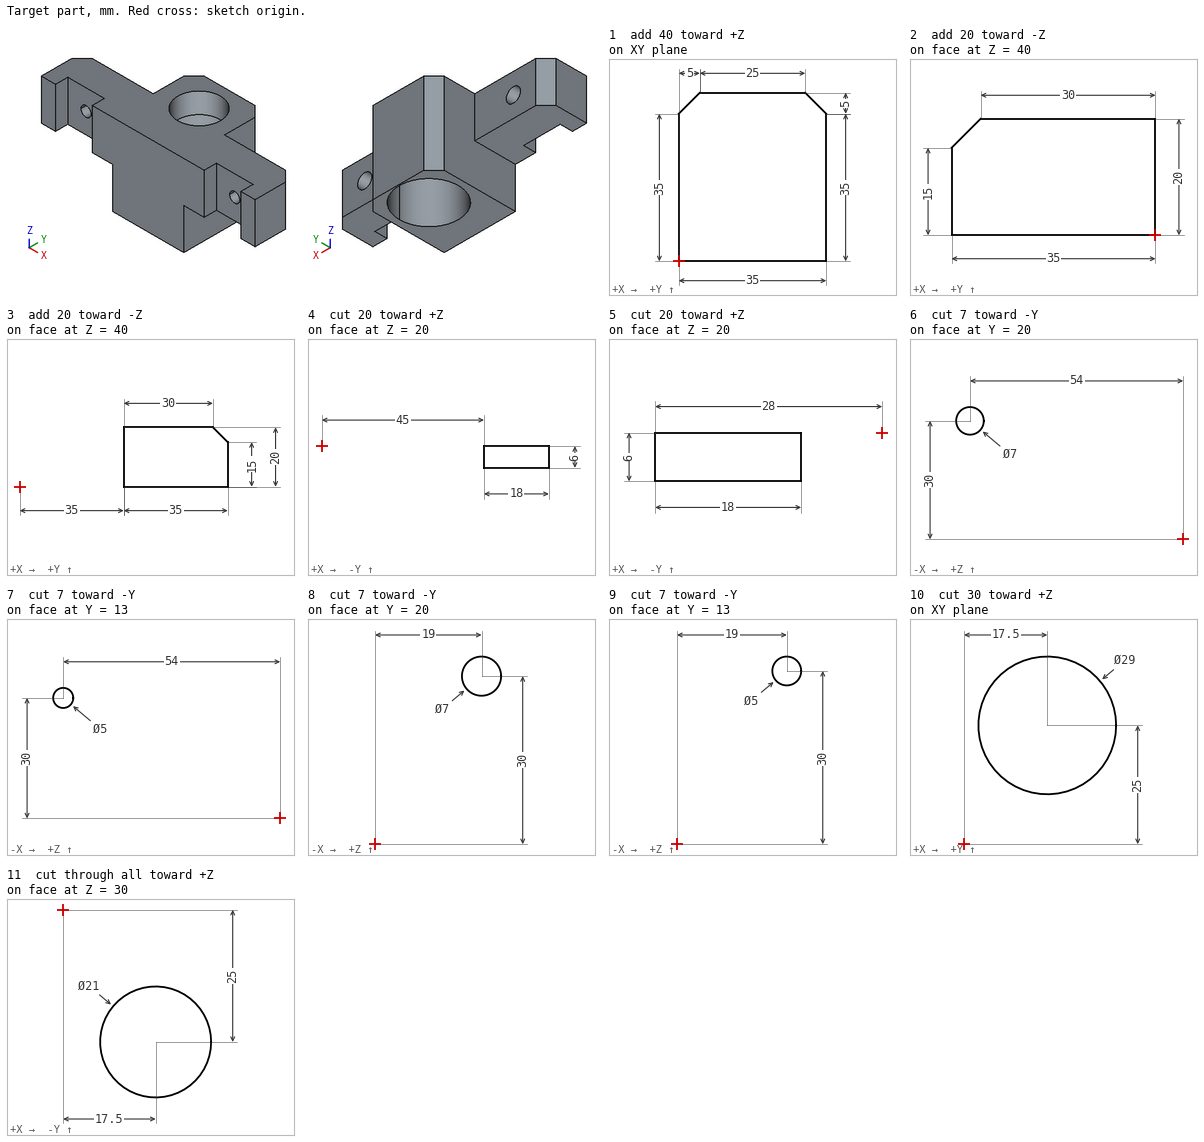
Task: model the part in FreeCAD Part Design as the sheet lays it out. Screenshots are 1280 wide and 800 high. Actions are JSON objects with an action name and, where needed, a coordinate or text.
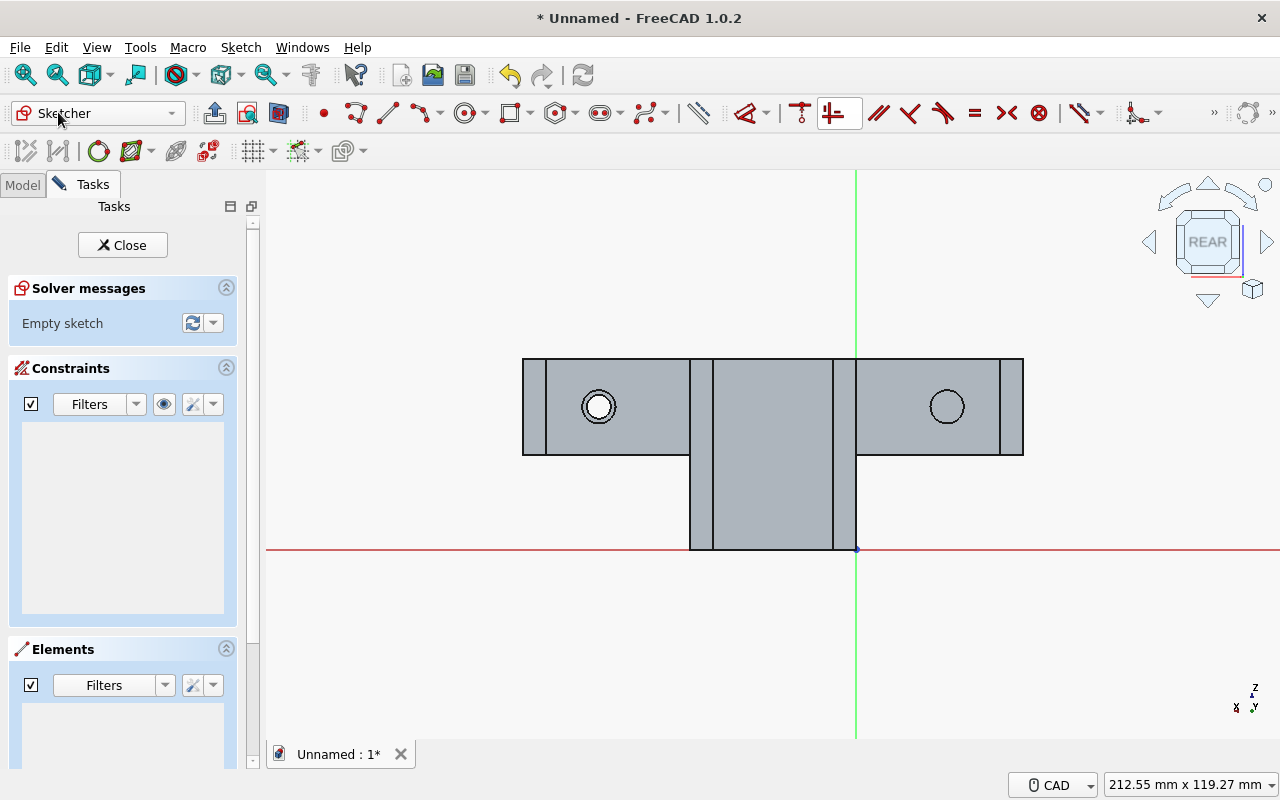
{"action": "left_click", "coordinate": [280, 114]}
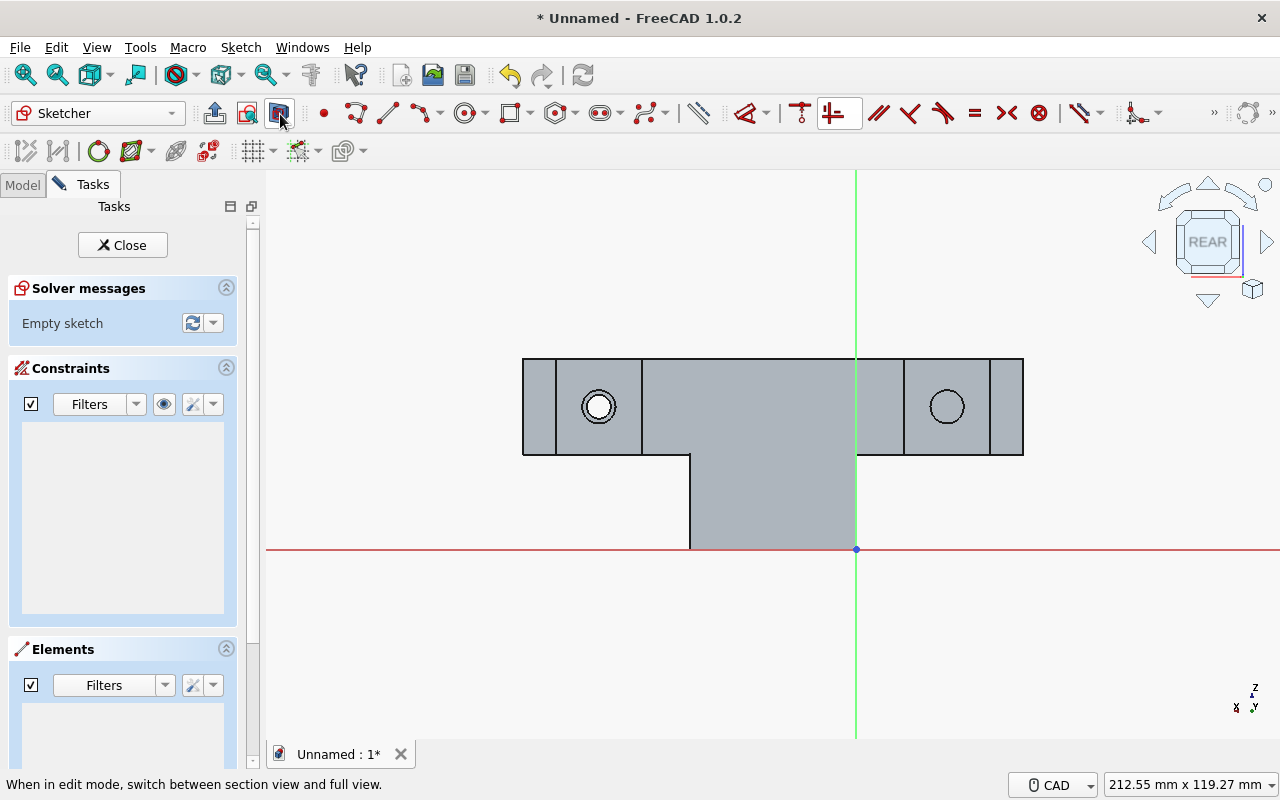
{"action": "scroll", "coordinate": [963, 404], "scroll_direction": "up", "scroll_amount": 14}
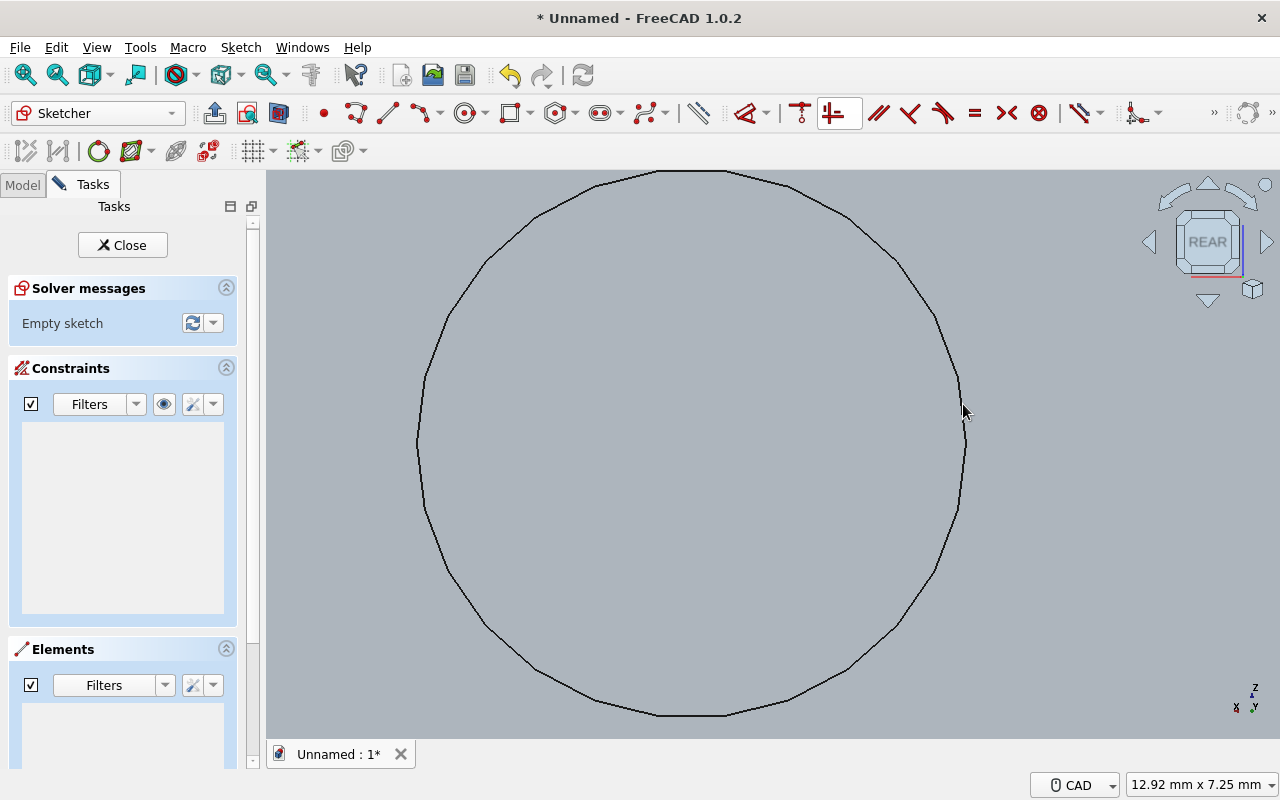
{"action": "left_click", "coordinate": [466, 114]}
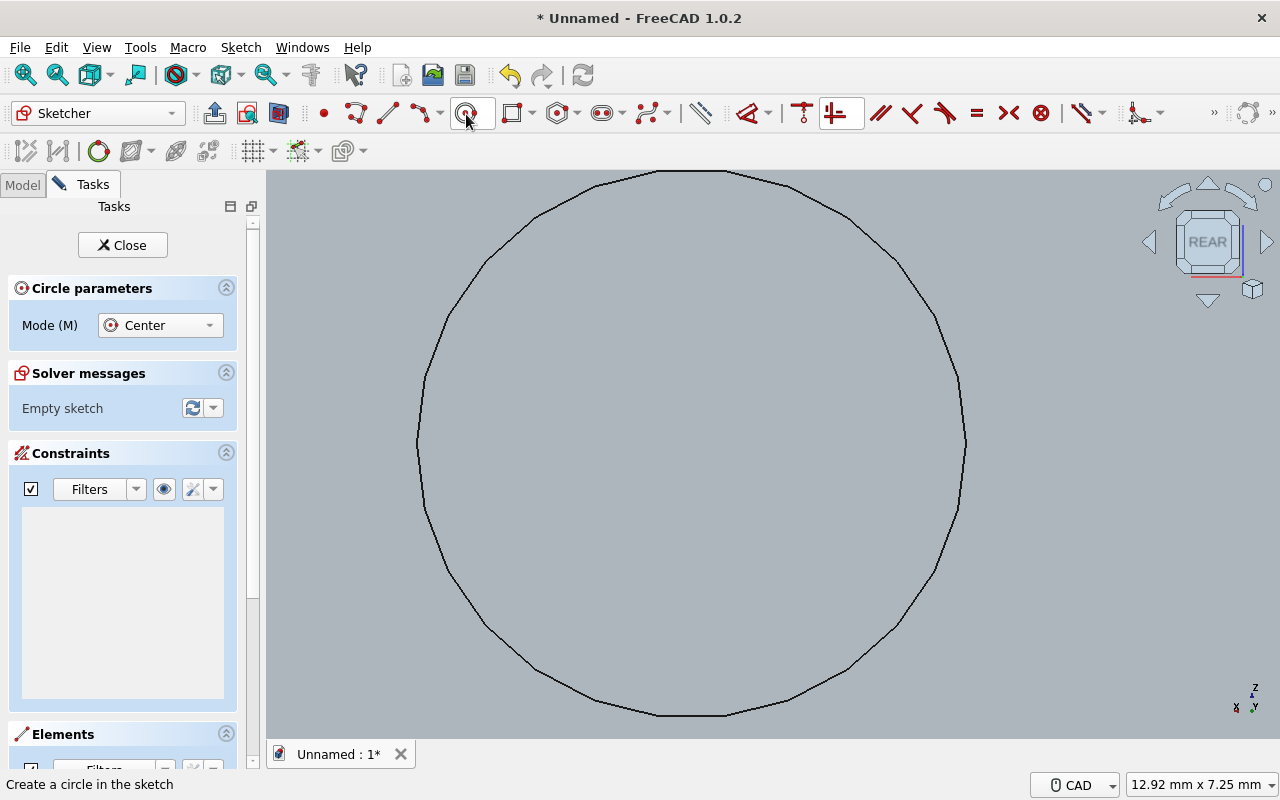
{"action": "left_click", "coordinate": [691, 444]}
{"action": "left_click", "coordinate": [830, 305]}
{"action": "key", "text": "Escape"}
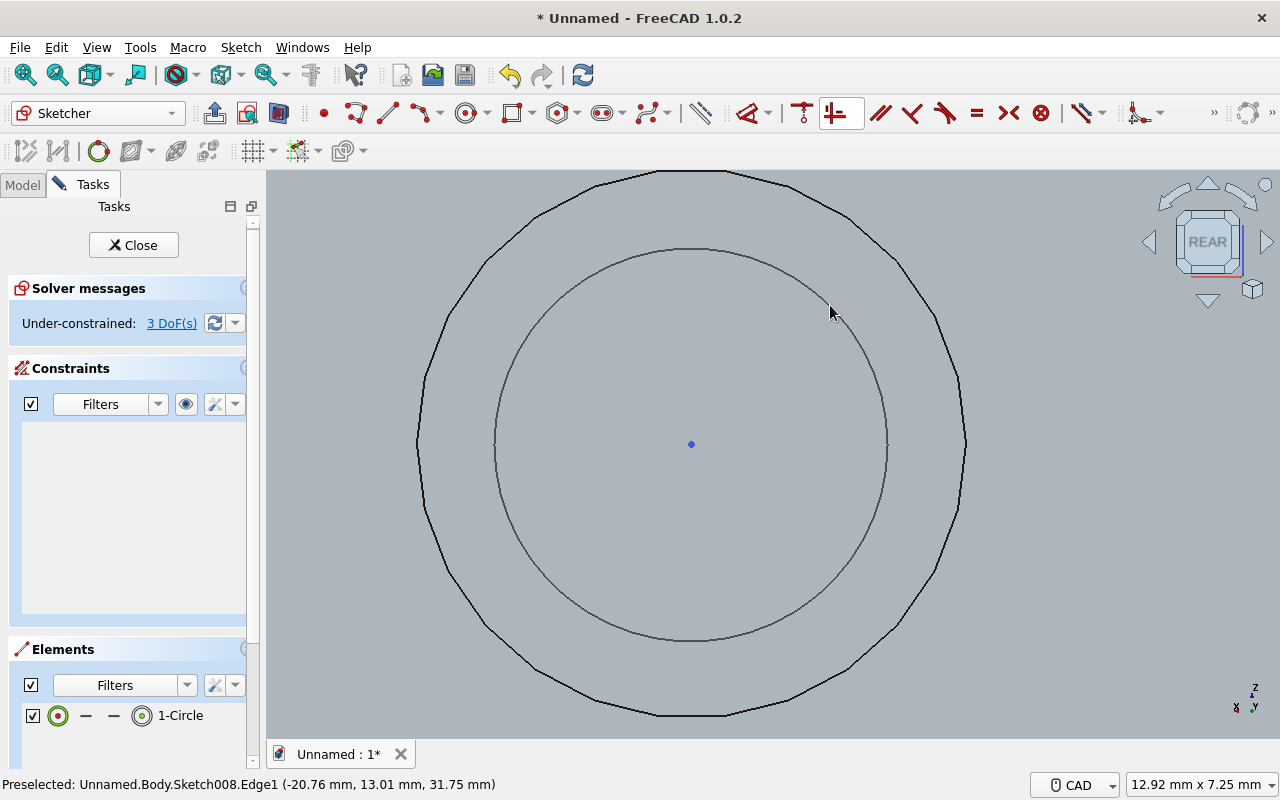
{"action": "left_click", "coordinate": [748, 114]}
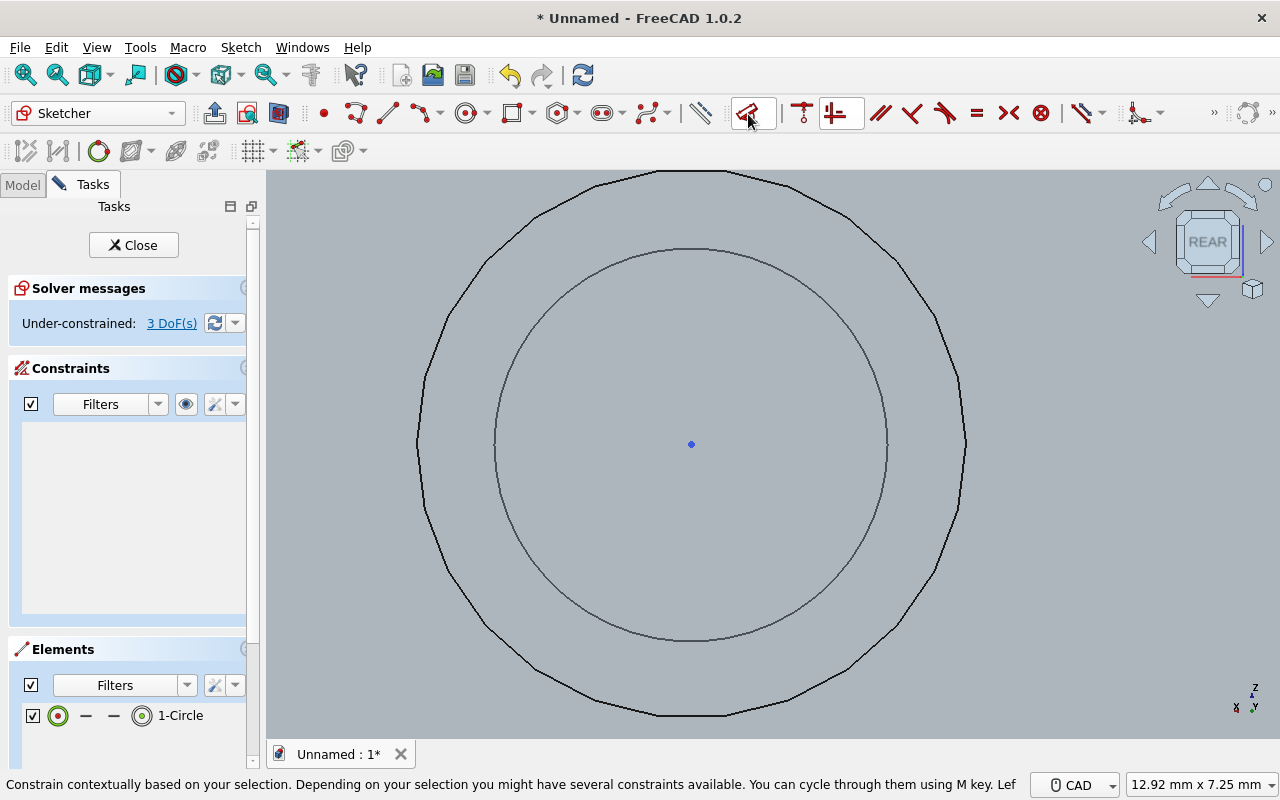
{"action": "left_click", "coordinate": [830, 306]}
{"action": "left_click", "coordinate": [853, 283]}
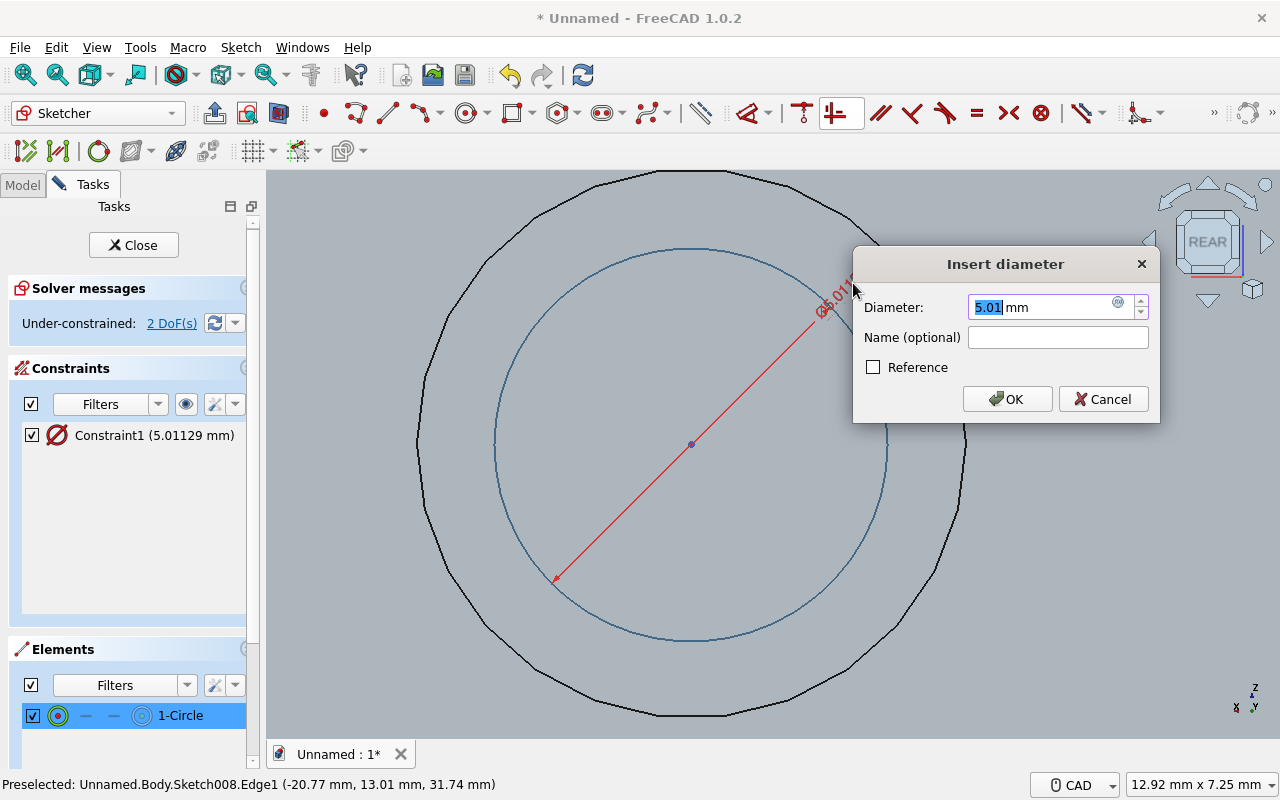
{"action": "type", "text": "5"}
{"action": "key", "text": "Return"}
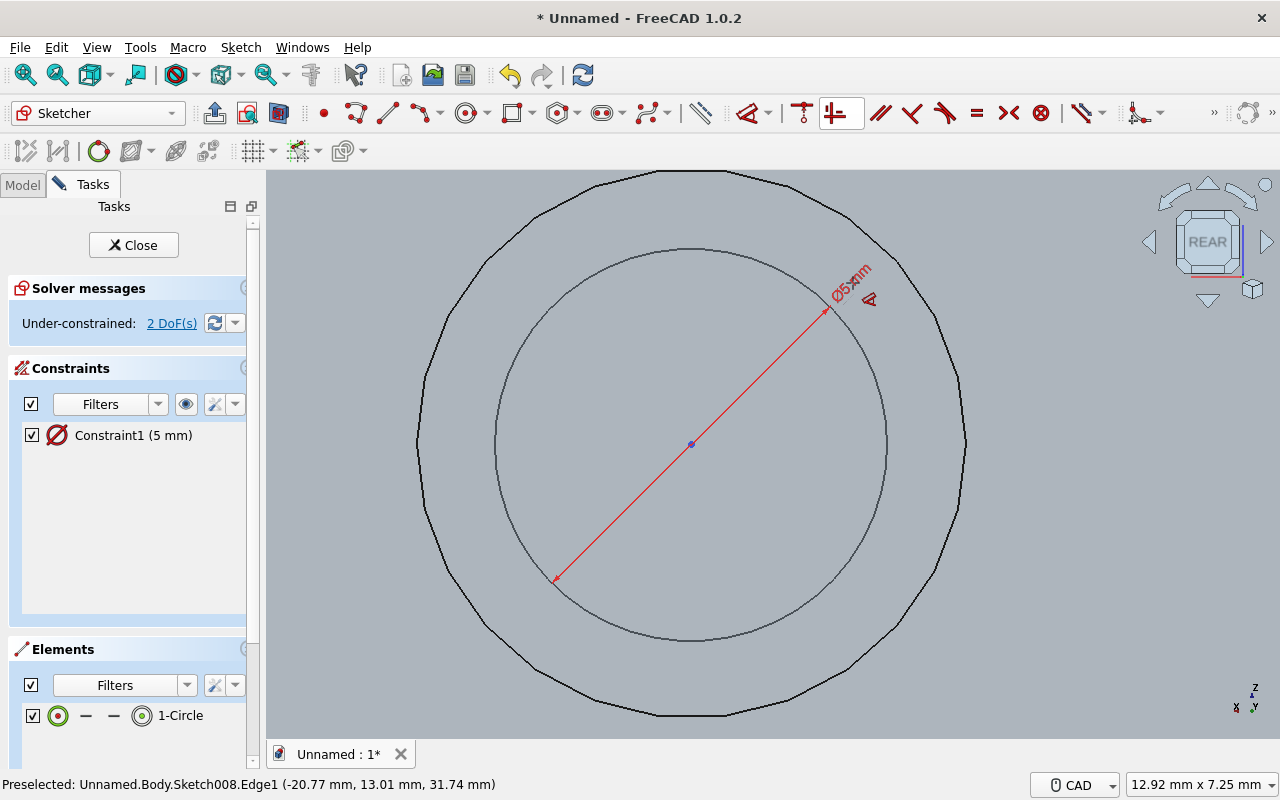
{"action": "left_click", "coordinate": [691, 445]}
{"action": "left_click", "coordinate": [401, 411]}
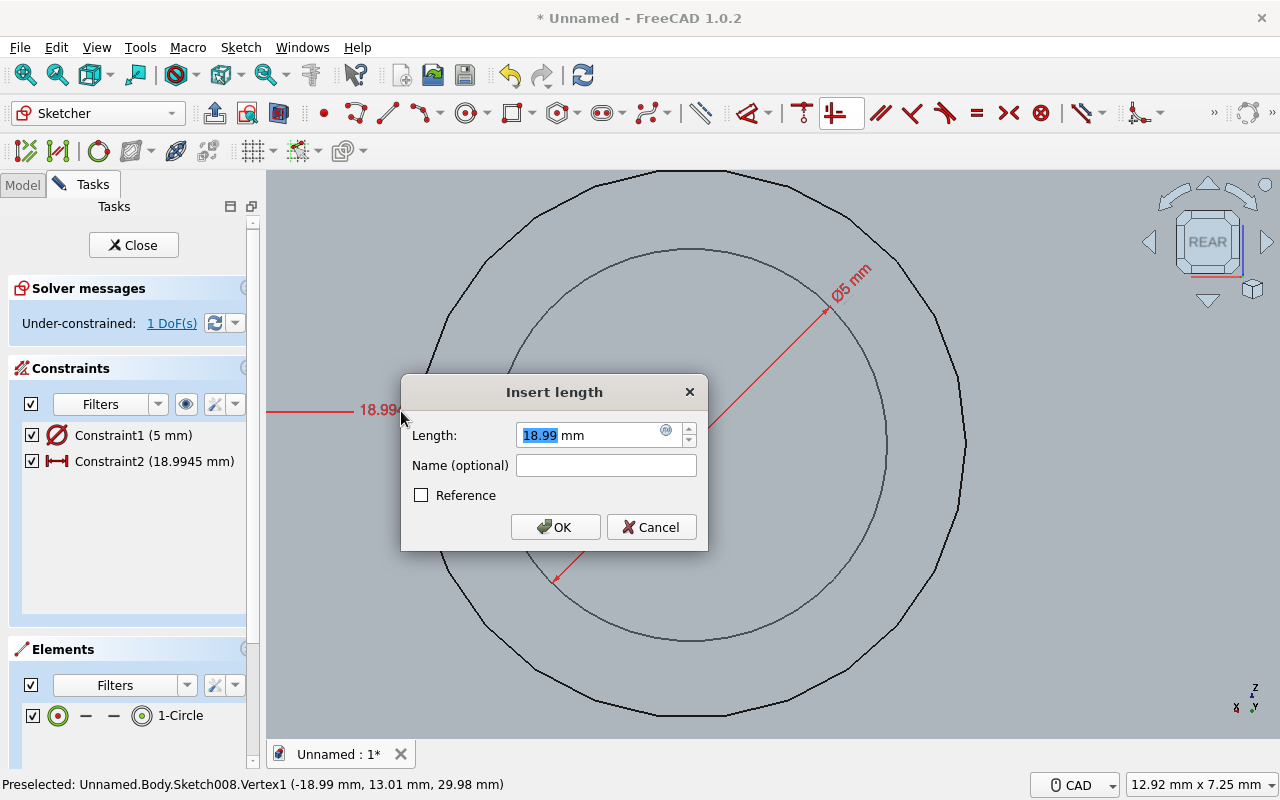
{"action": "type", "text": "19"}
{"action": "key", "text": "Return"}